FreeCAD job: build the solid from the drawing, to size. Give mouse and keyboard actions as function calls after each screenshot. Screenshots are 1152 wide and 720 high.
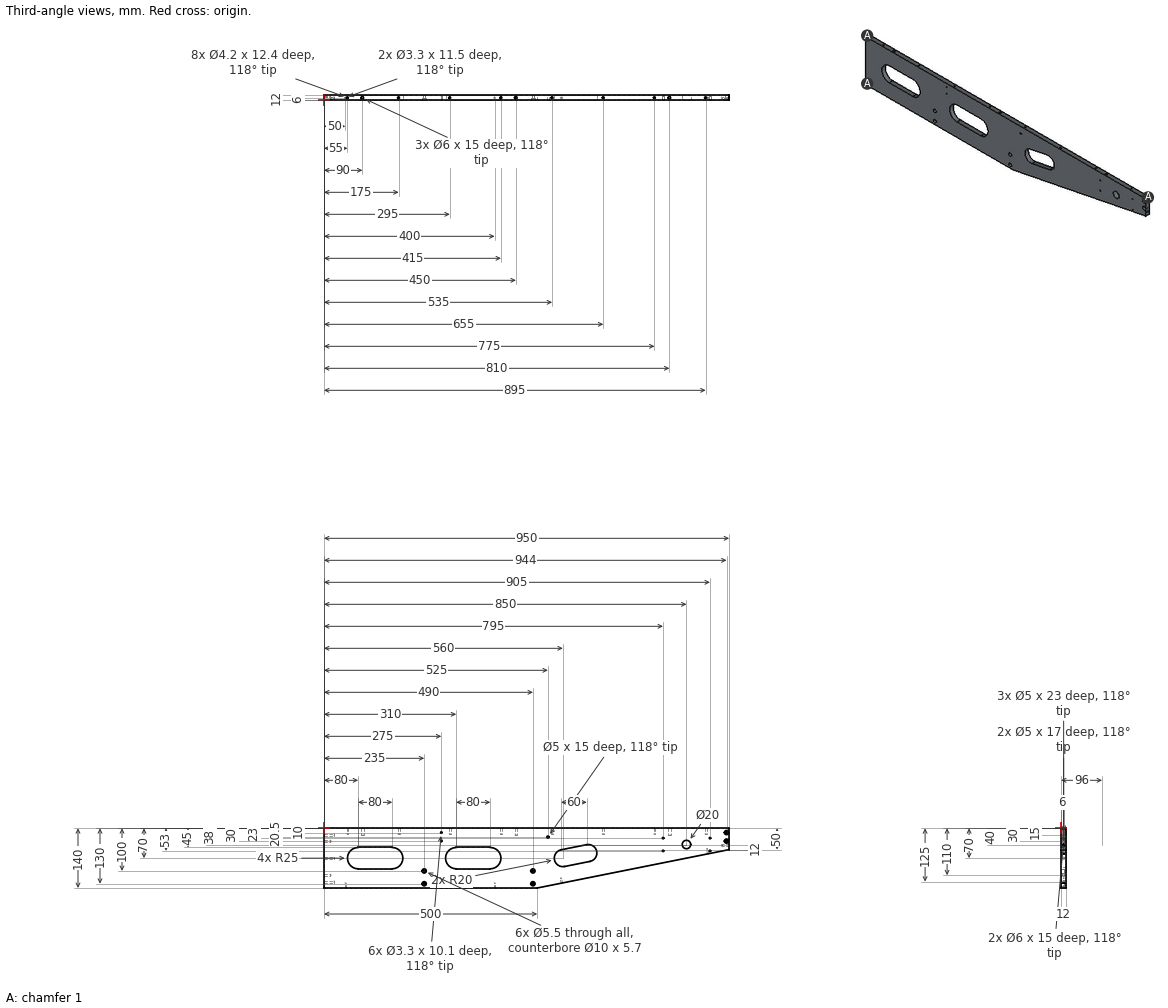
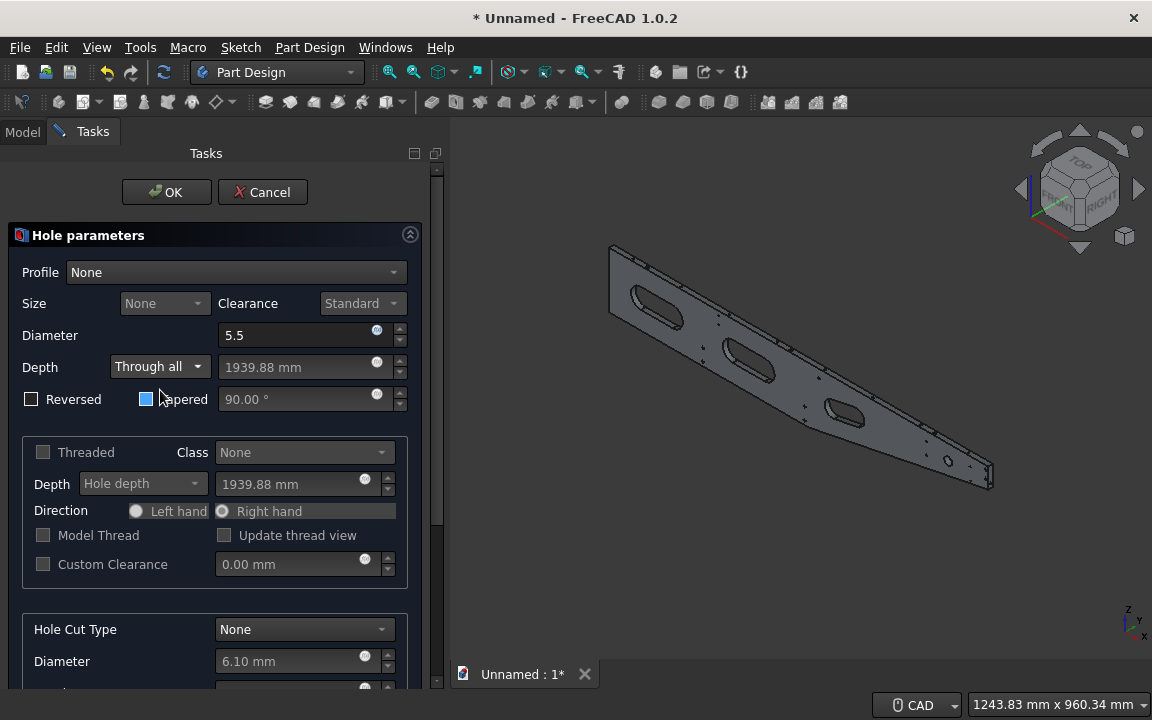
click(306, 630)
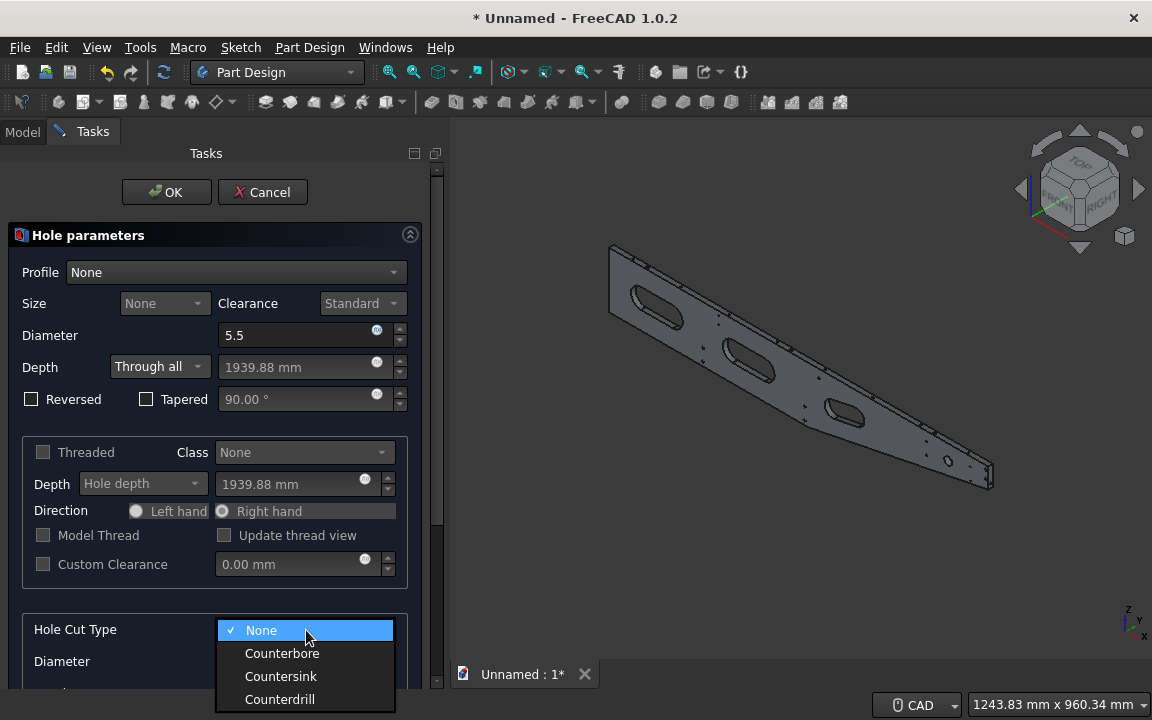
click(304, 654)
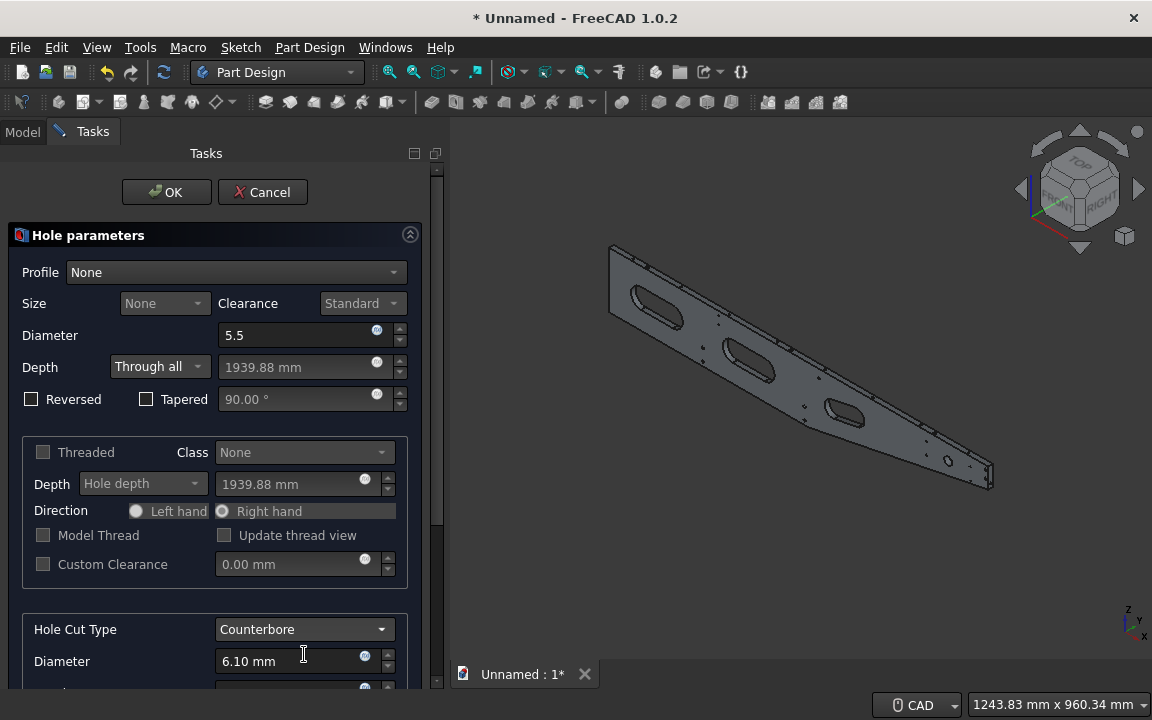
triple_click(298, 661)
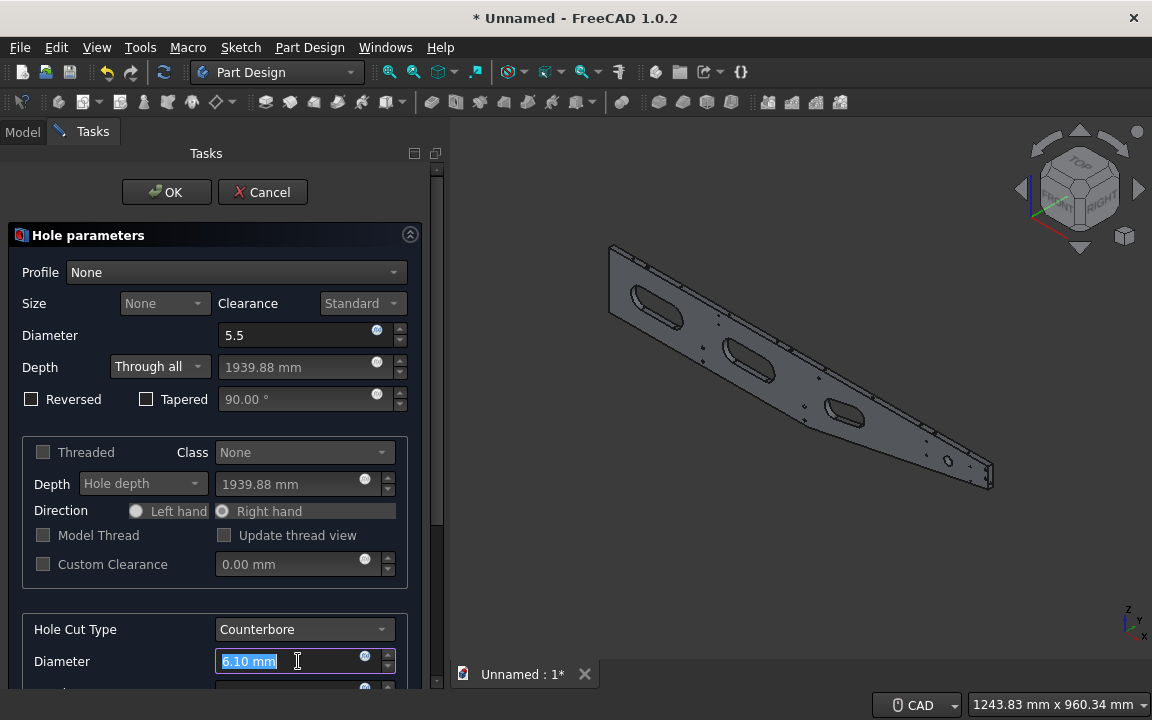
text(10)
key(Tab)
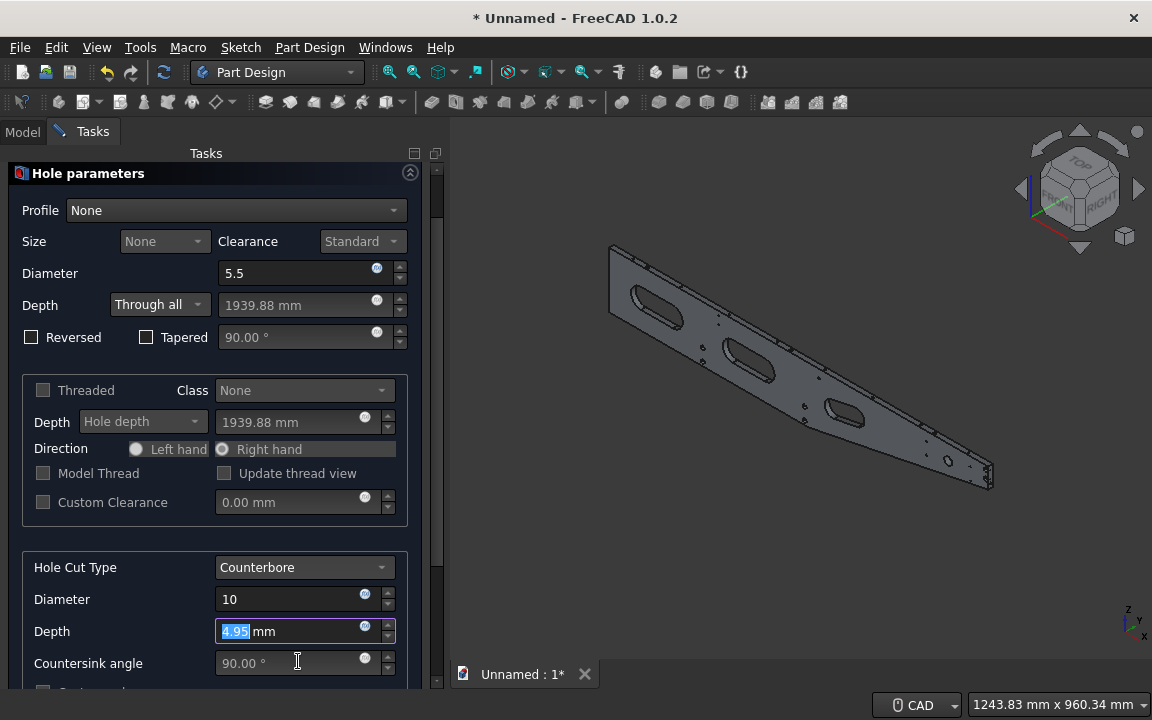
text(5.7)
key(Tab)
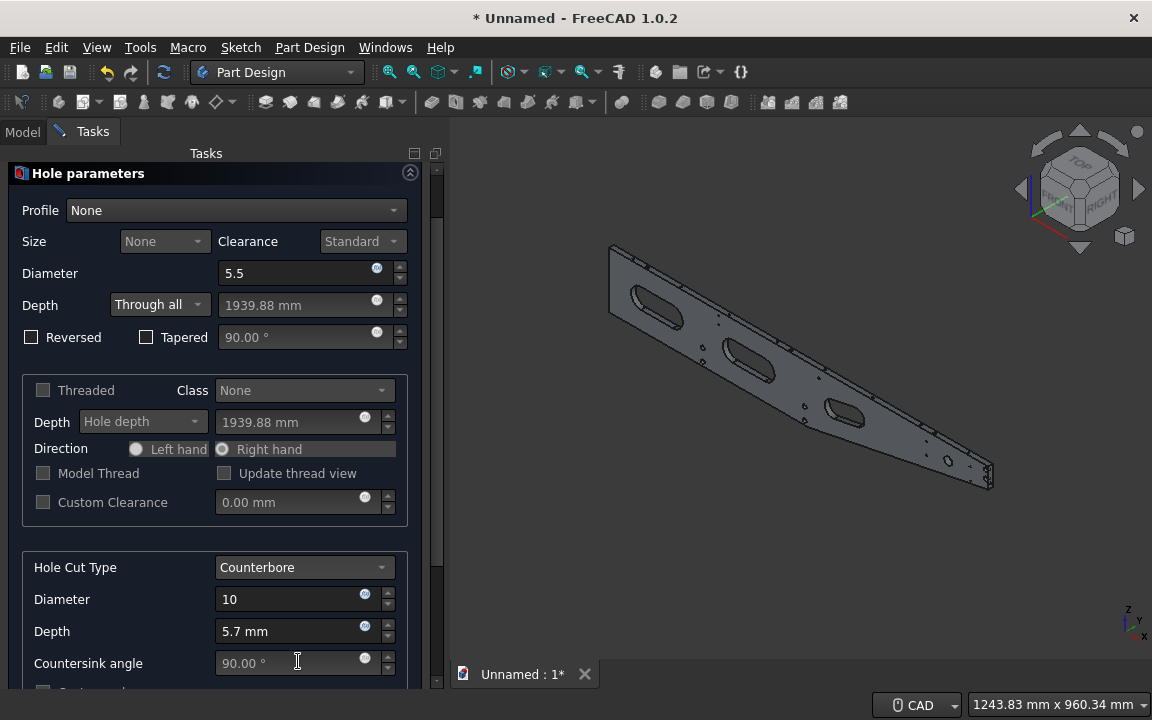
scroll(437, 426, up, 2)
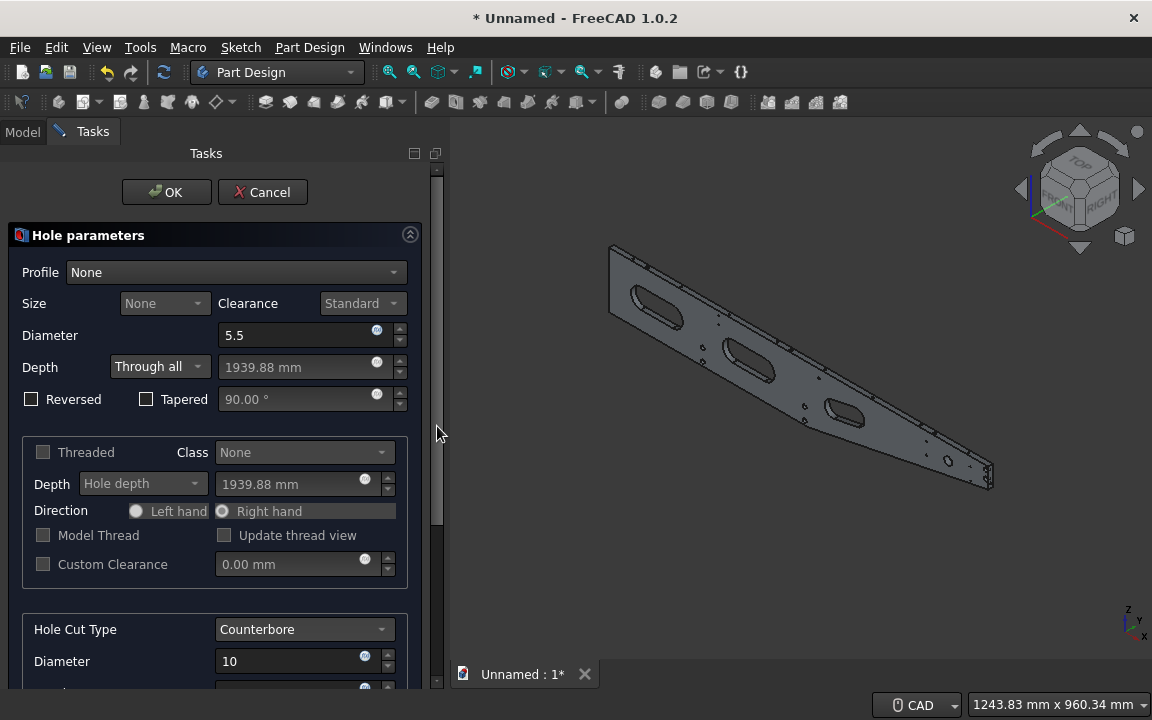
click(167, 192)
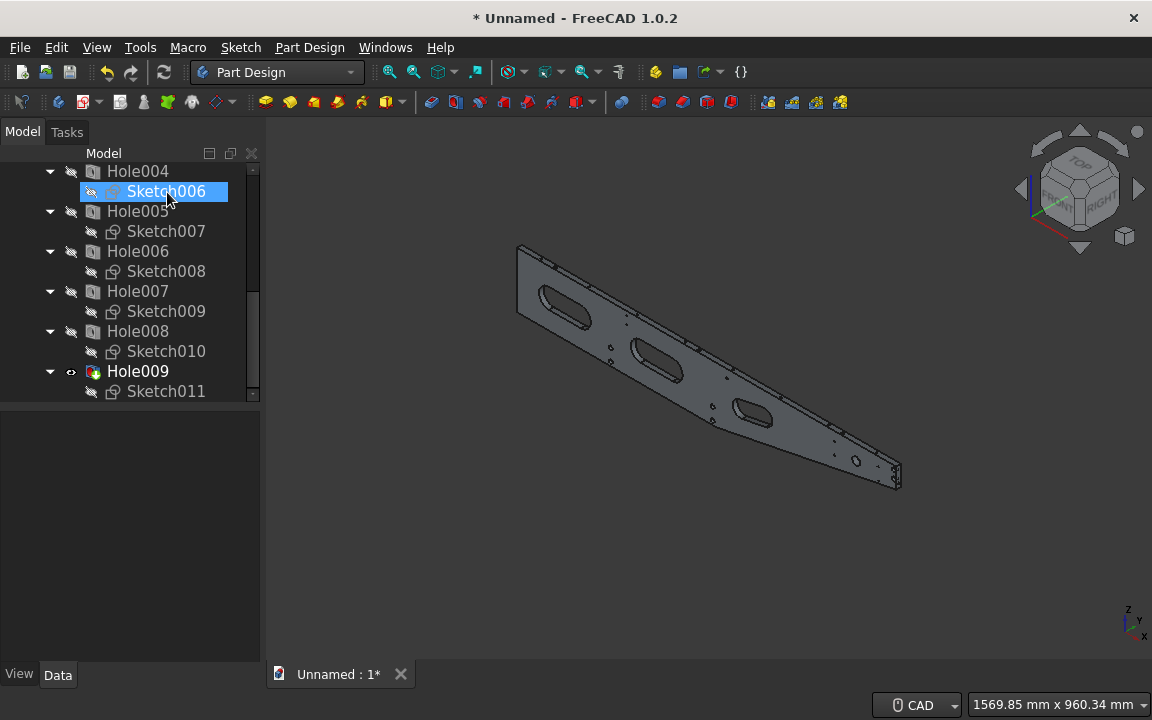
scroll(899, 464, up, 9)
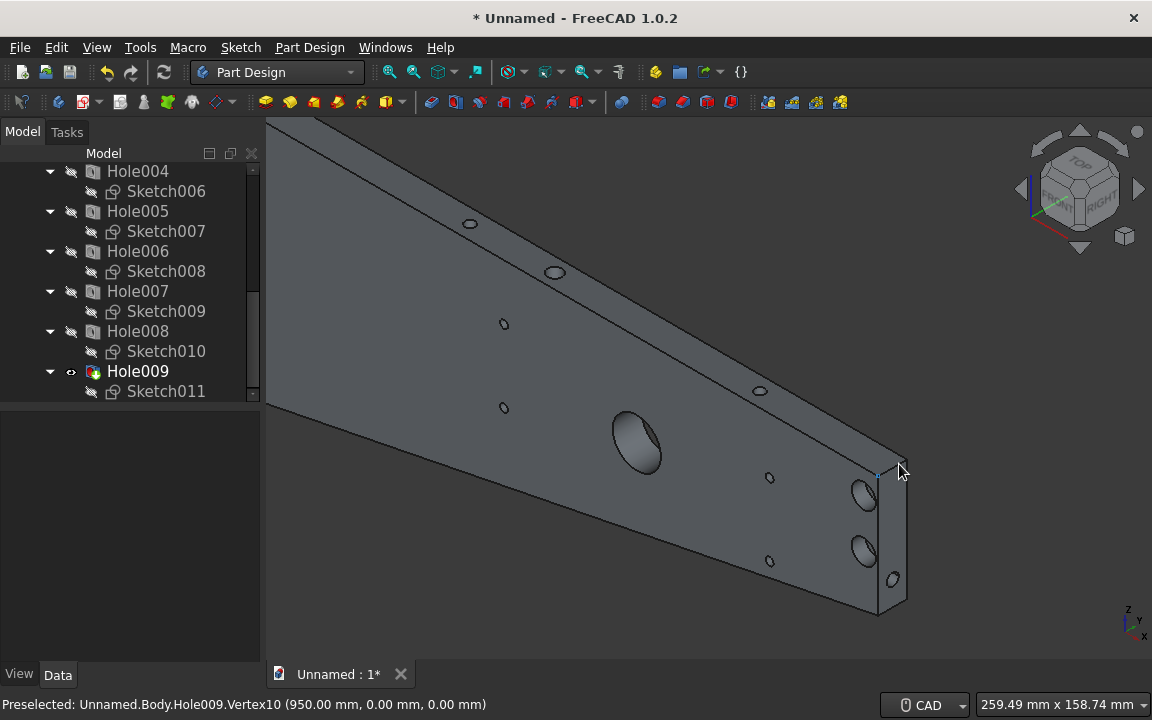
click(893, 467)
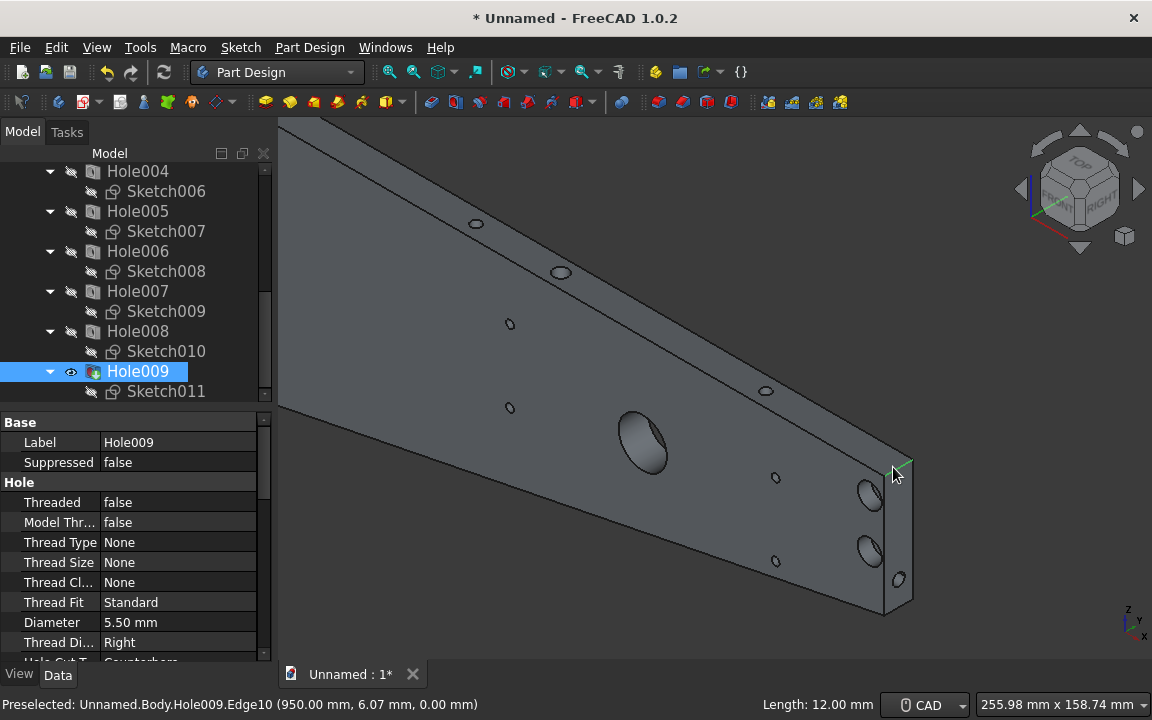
key(v)
key(f)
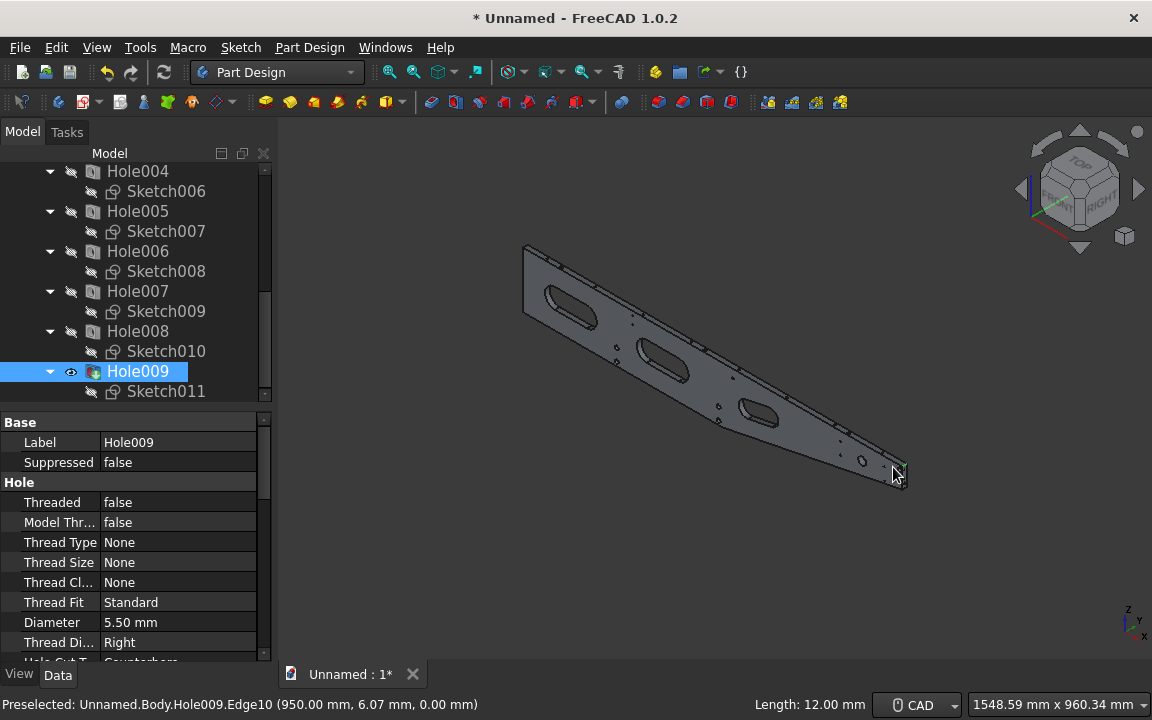
key(2)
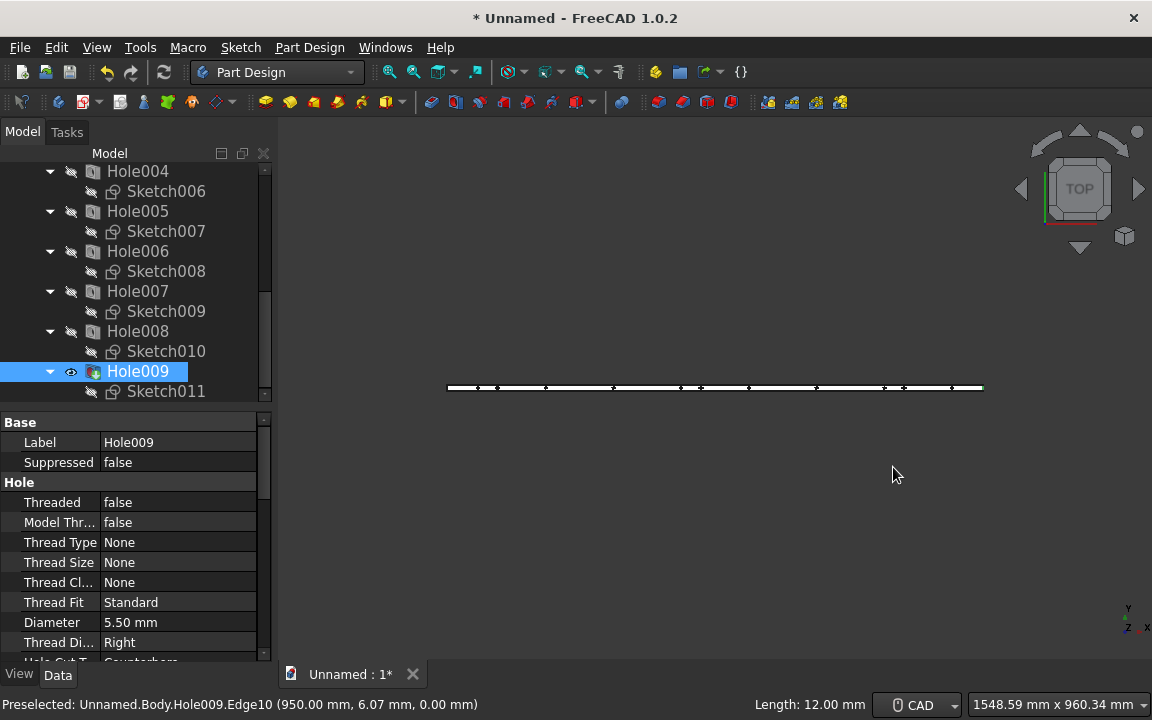
scroll(447, 387, up, 9)